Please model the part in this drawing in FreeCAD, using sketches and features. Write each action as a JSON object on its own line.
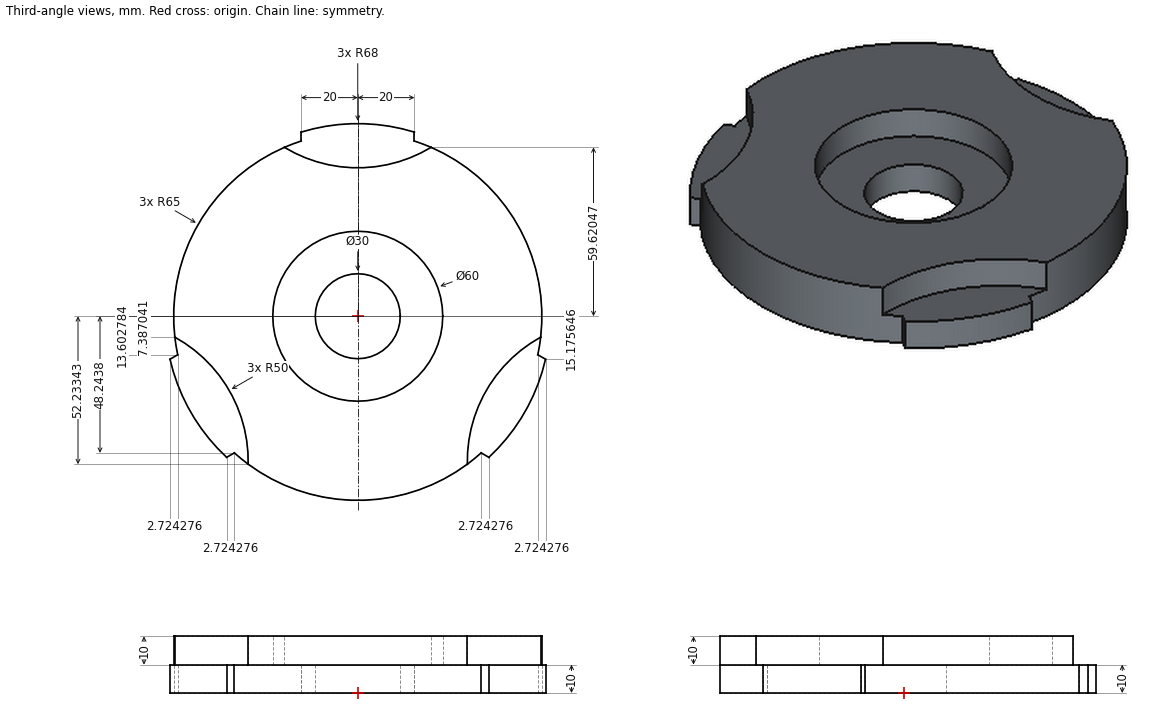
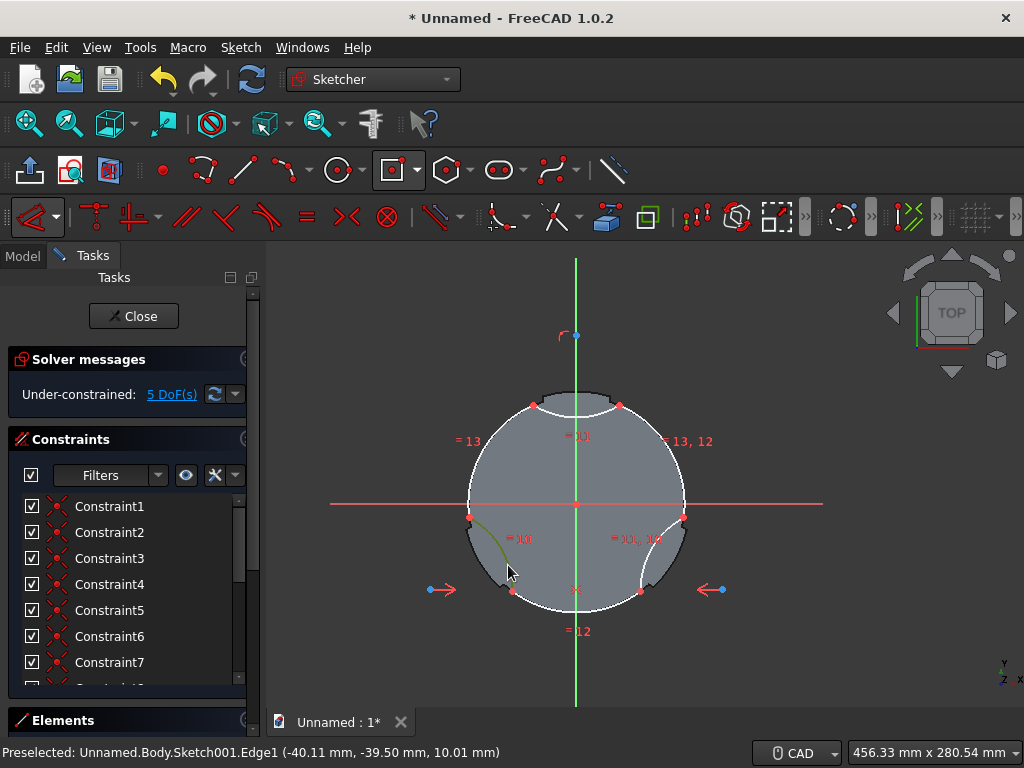
{"action": "left_click", "coordinate": [58, 218]}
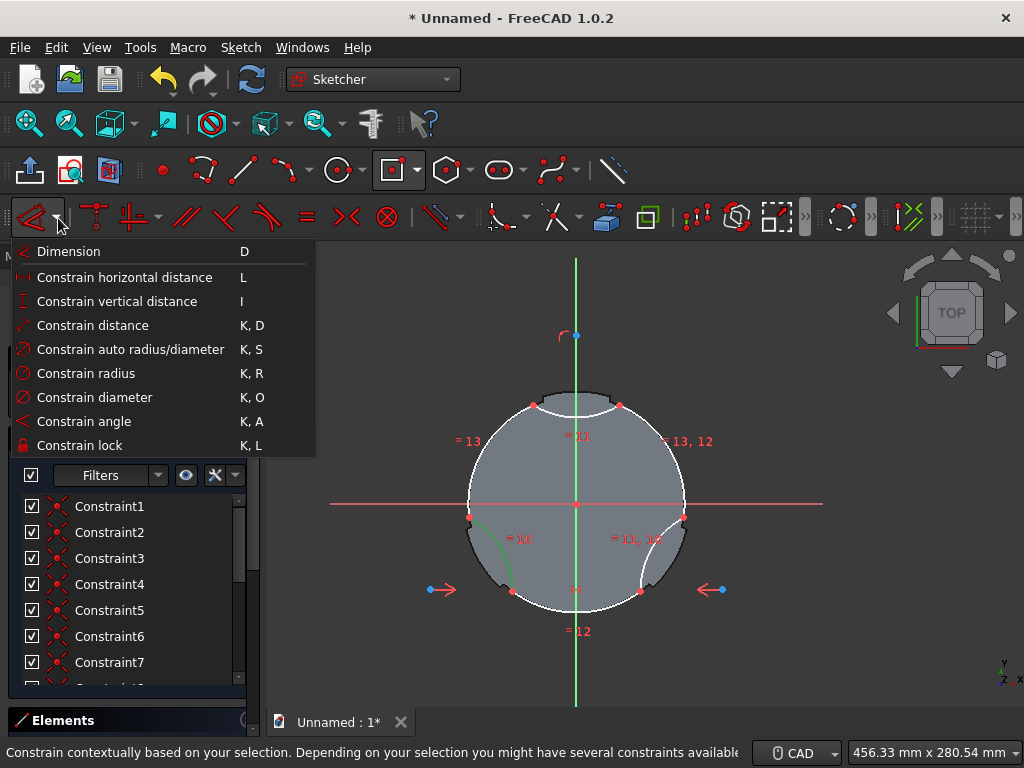
{"action": "left_click", "coordinate": [164, 373]}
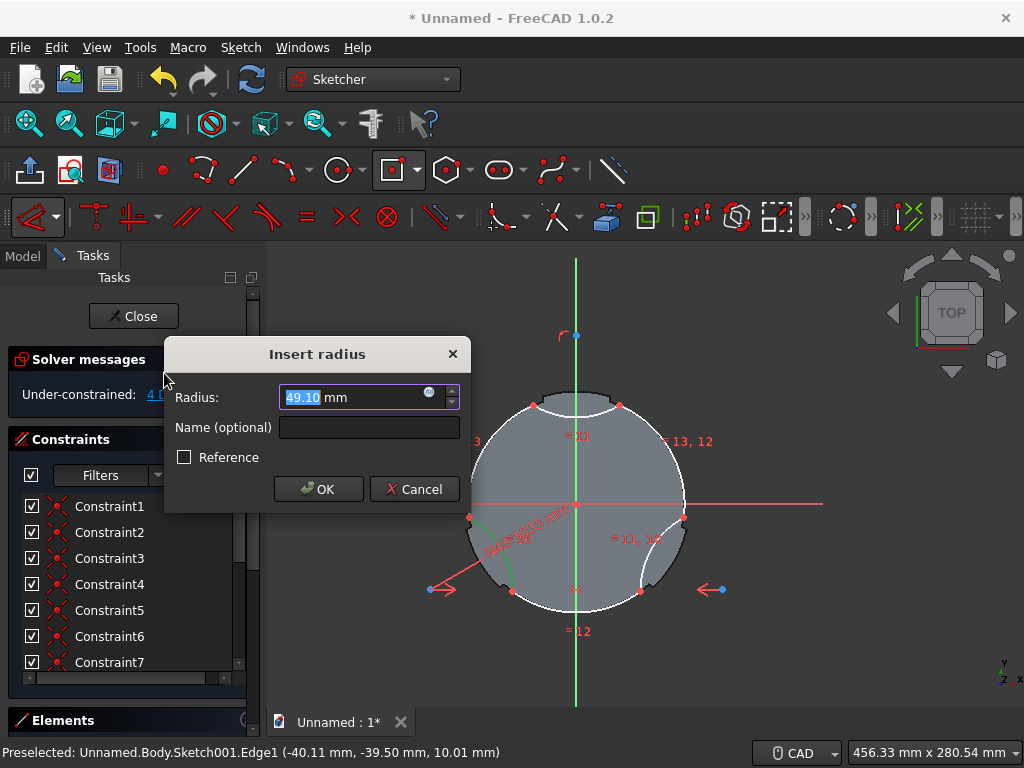
{"action": "type", "text": "50"}
{"action": "key", "text": "Return"}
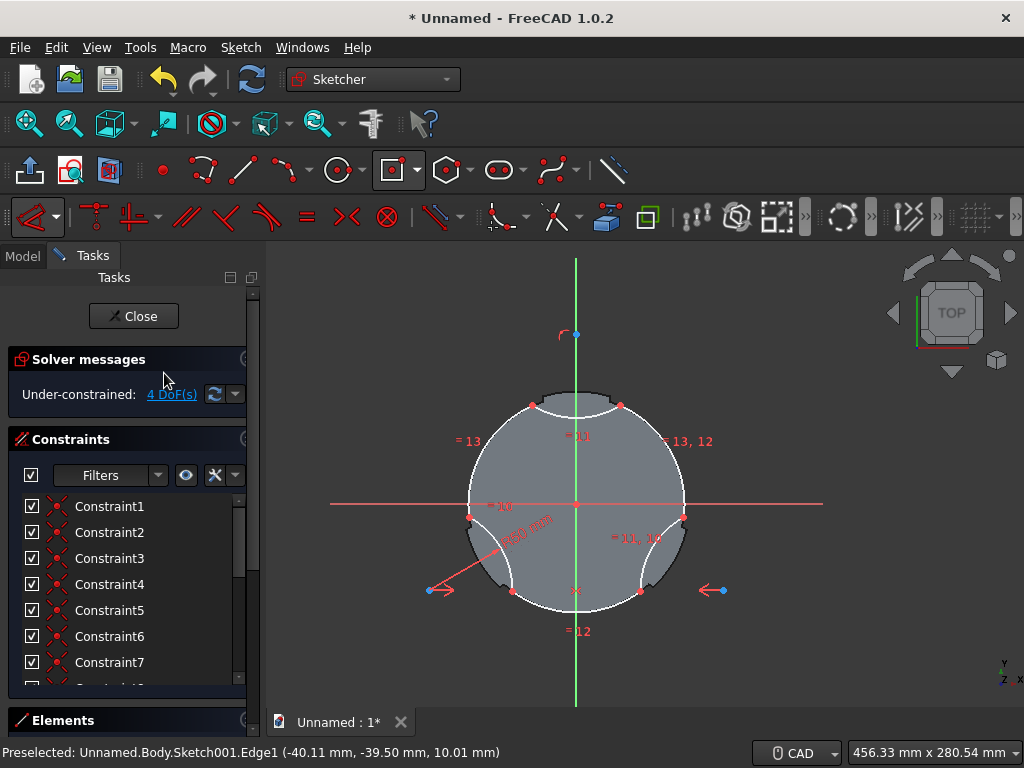
{"action": "left_click", "coordinate": [549, 609]}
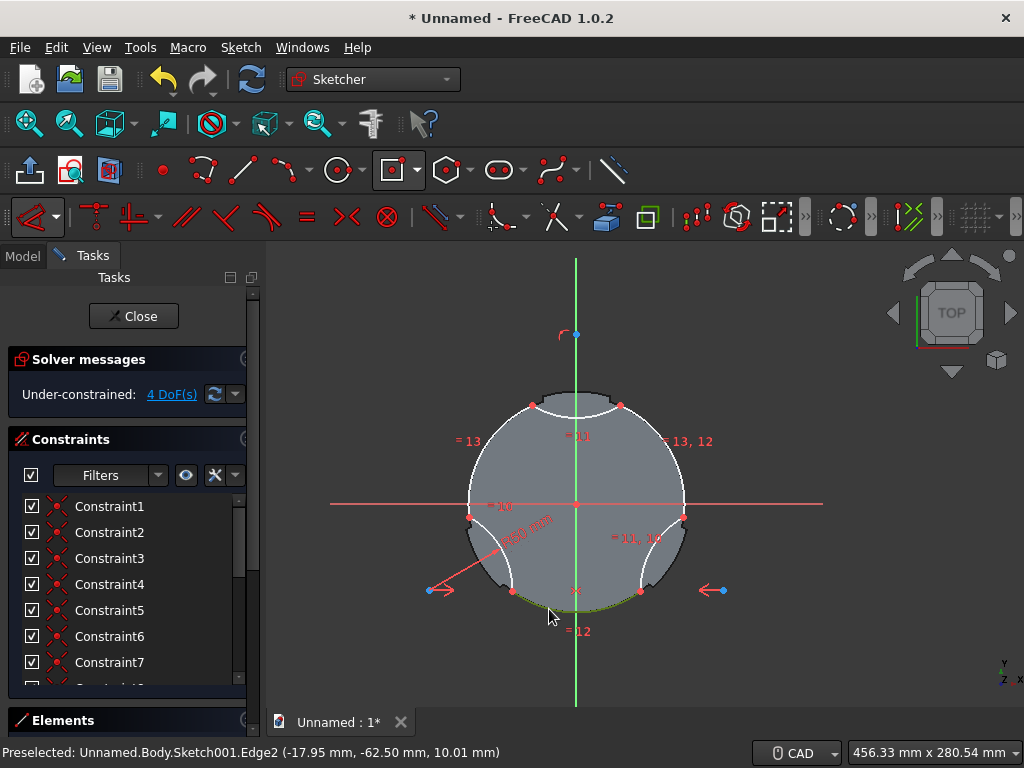
{"action": "key", "text": "k r"}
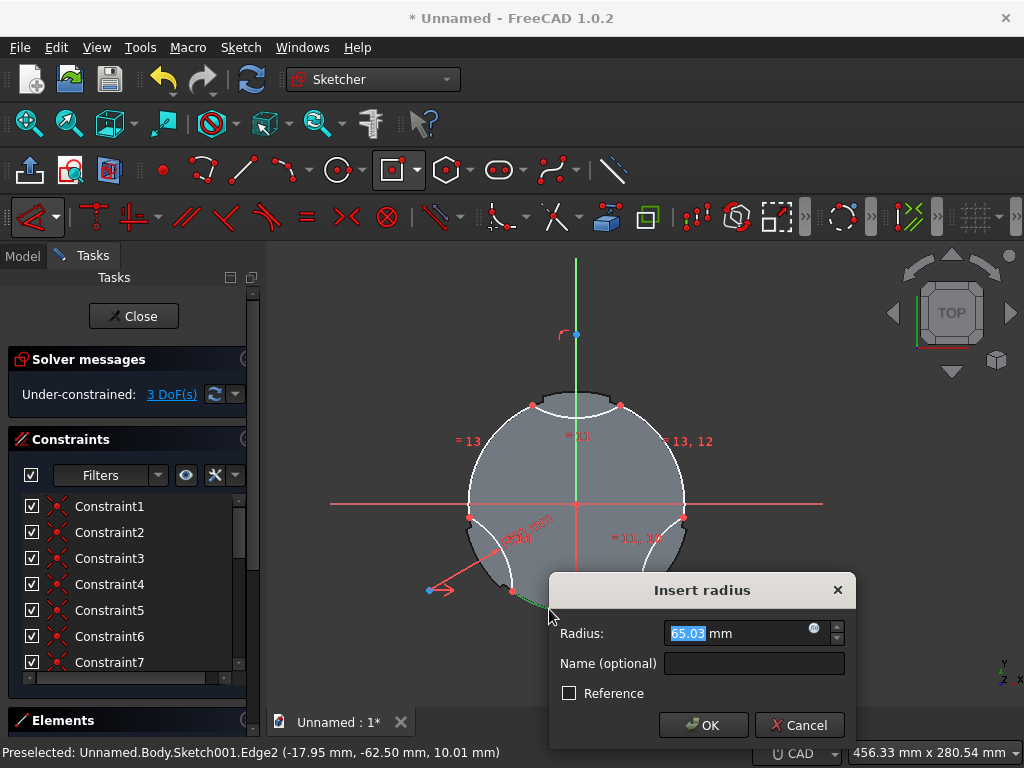
{"action": "type", "text": "65"}
{"action": "key", "text": "Return"}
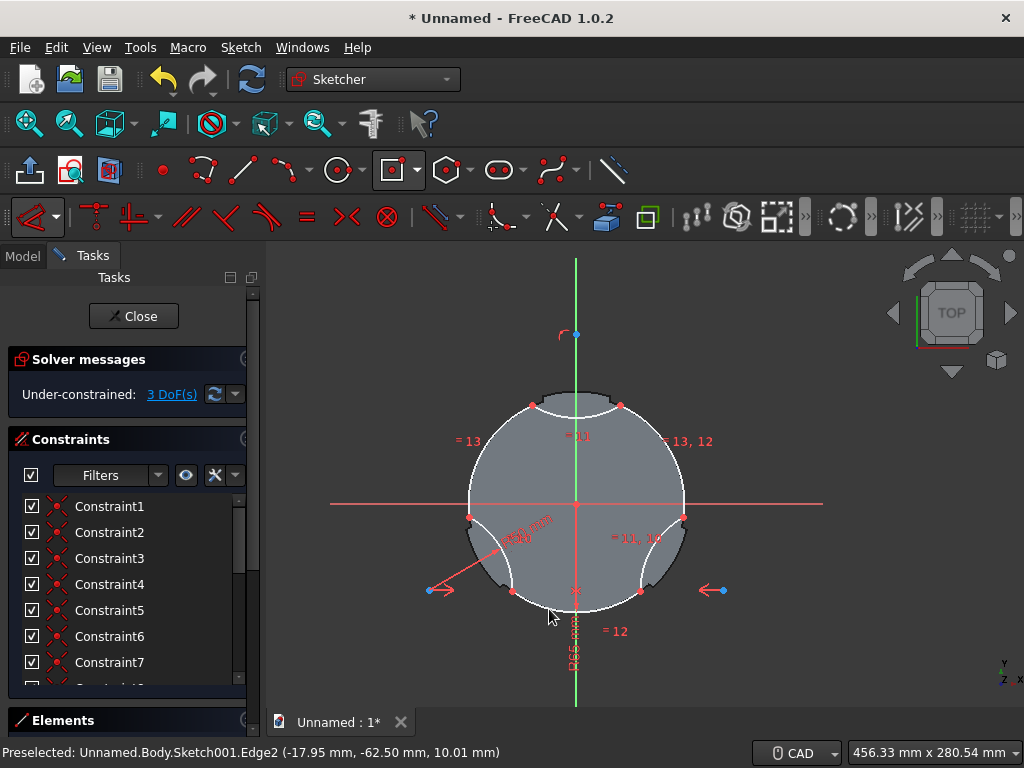
{"action": "left_click", "coordinate": [512, 591]}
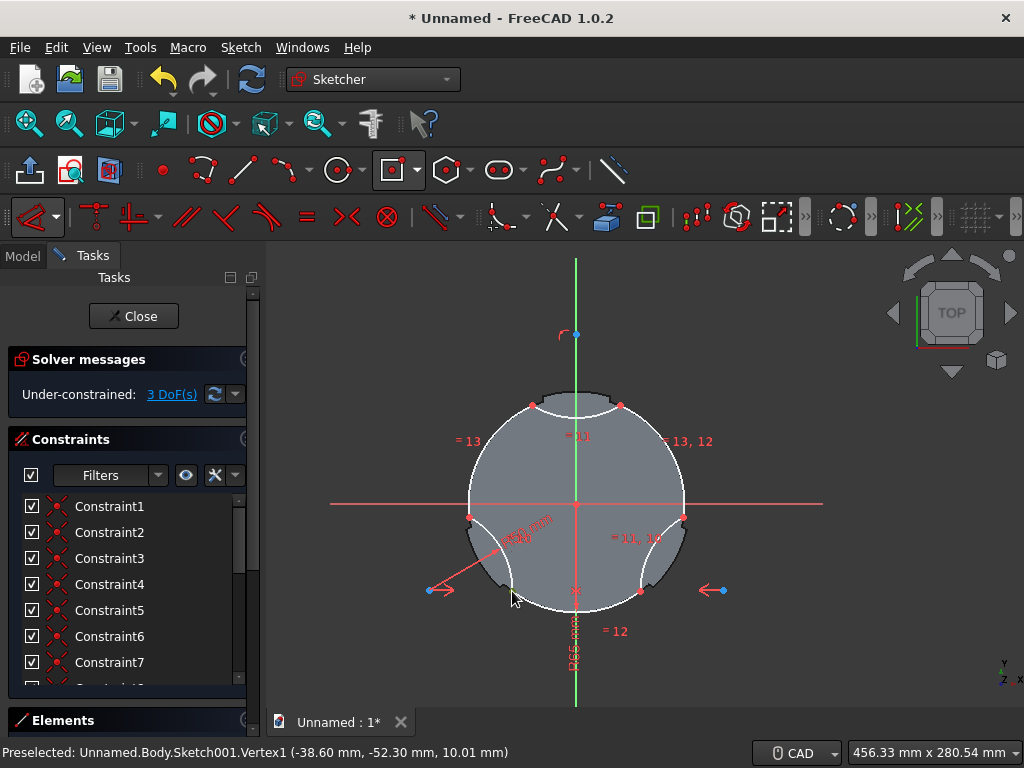
{"action": "key", "text": "i"}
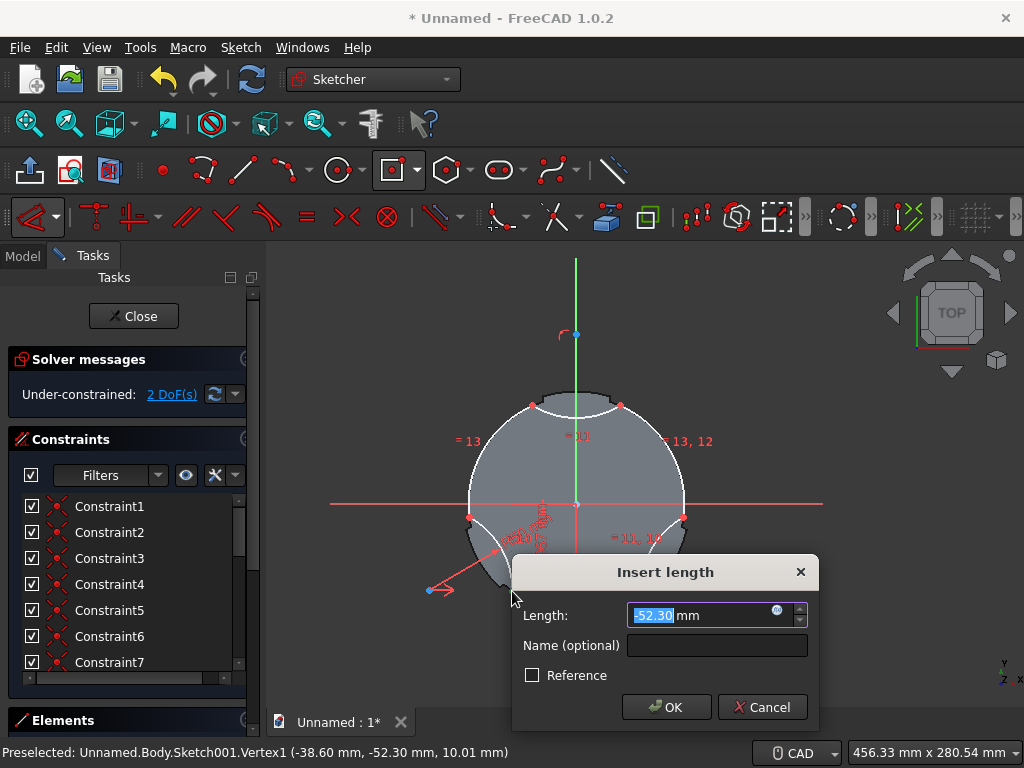
{"action": "type", "text": "-52.23343"}
{"action": "key", "text": "Return"}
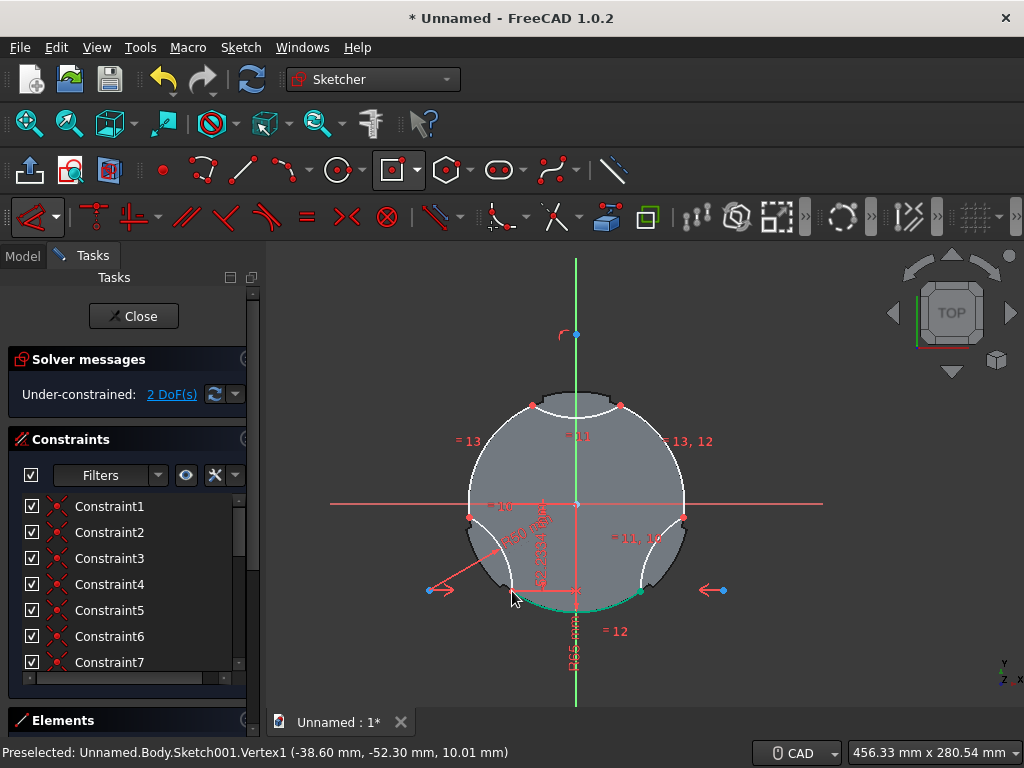
{"action": "scroll", "coordinate": [469, 517], "scroll_direction": "up", "scroll_amount": 6}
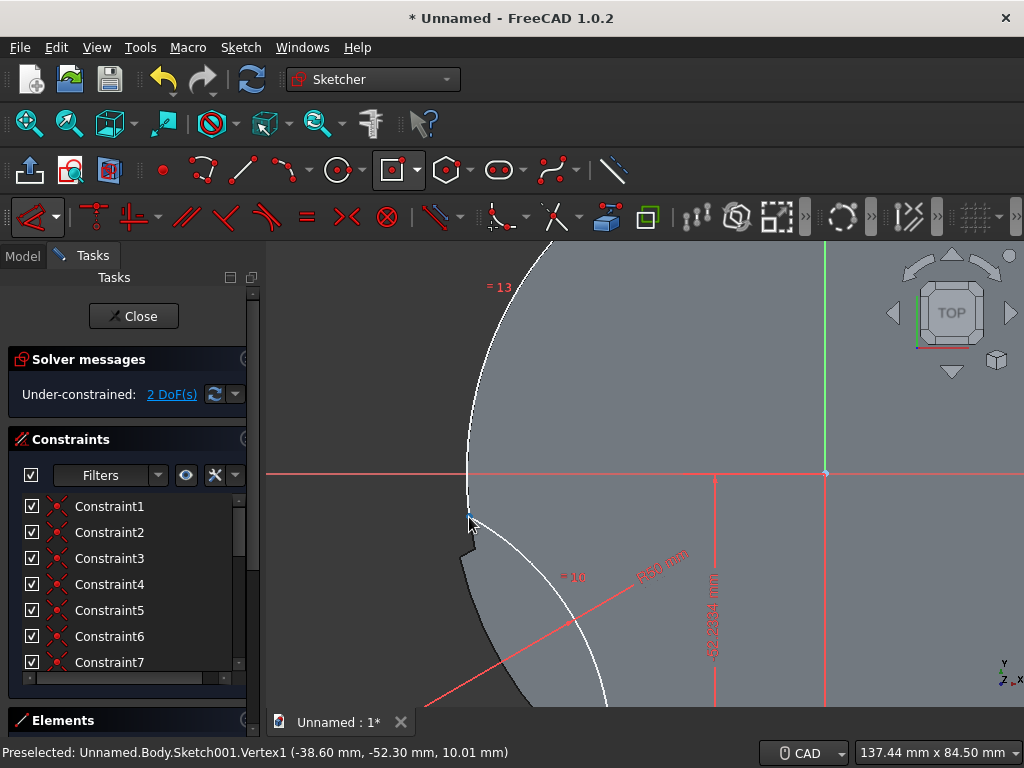
{"action": "left_click", "coordinate": [469, 517]}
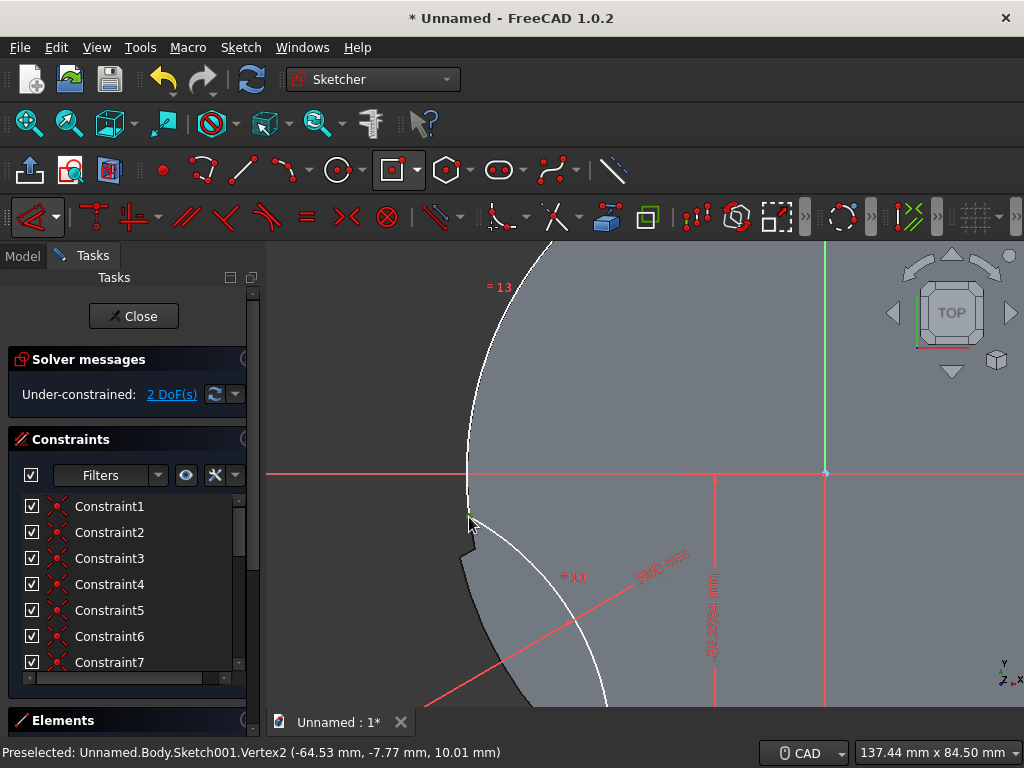
{"action": "key", "text": "i"}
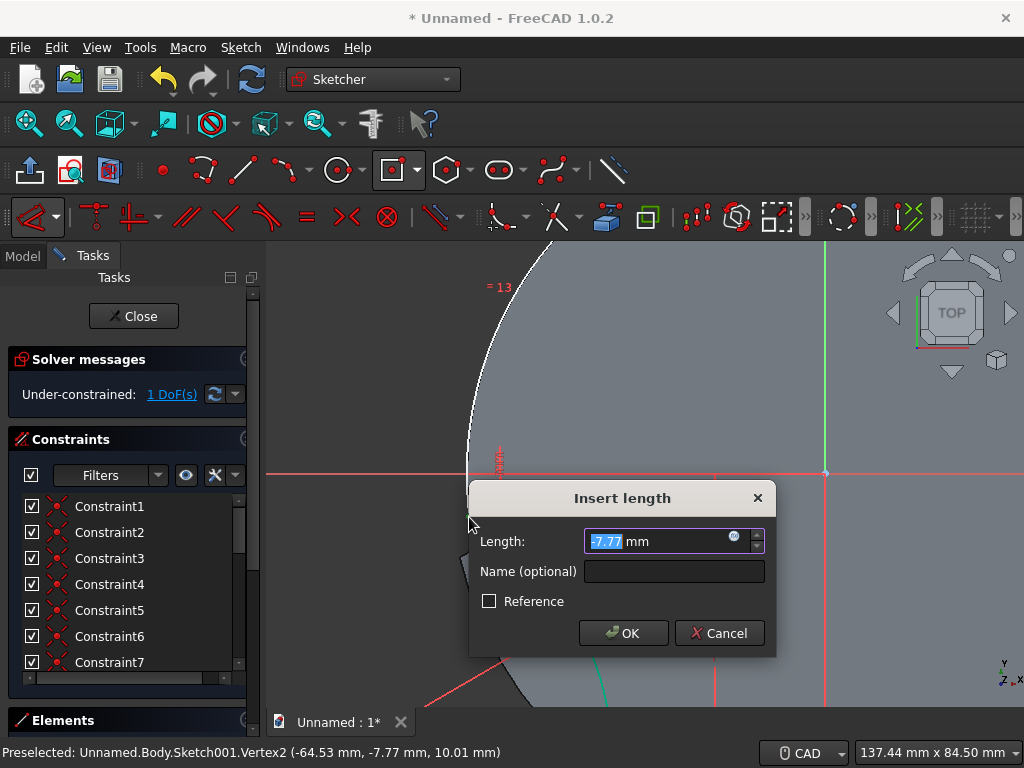
{"action": "type", "text": "-7.387041"}
{"action": "key", "text": "Return"}